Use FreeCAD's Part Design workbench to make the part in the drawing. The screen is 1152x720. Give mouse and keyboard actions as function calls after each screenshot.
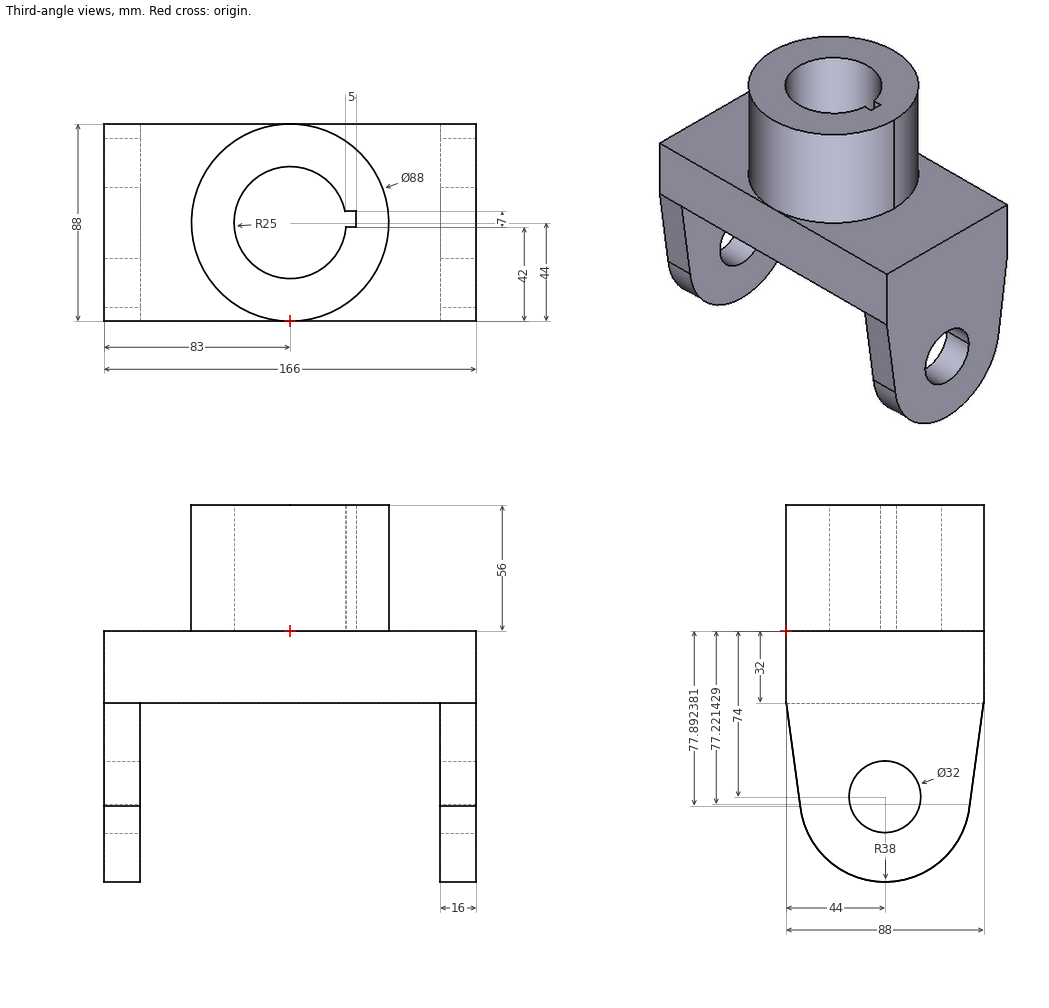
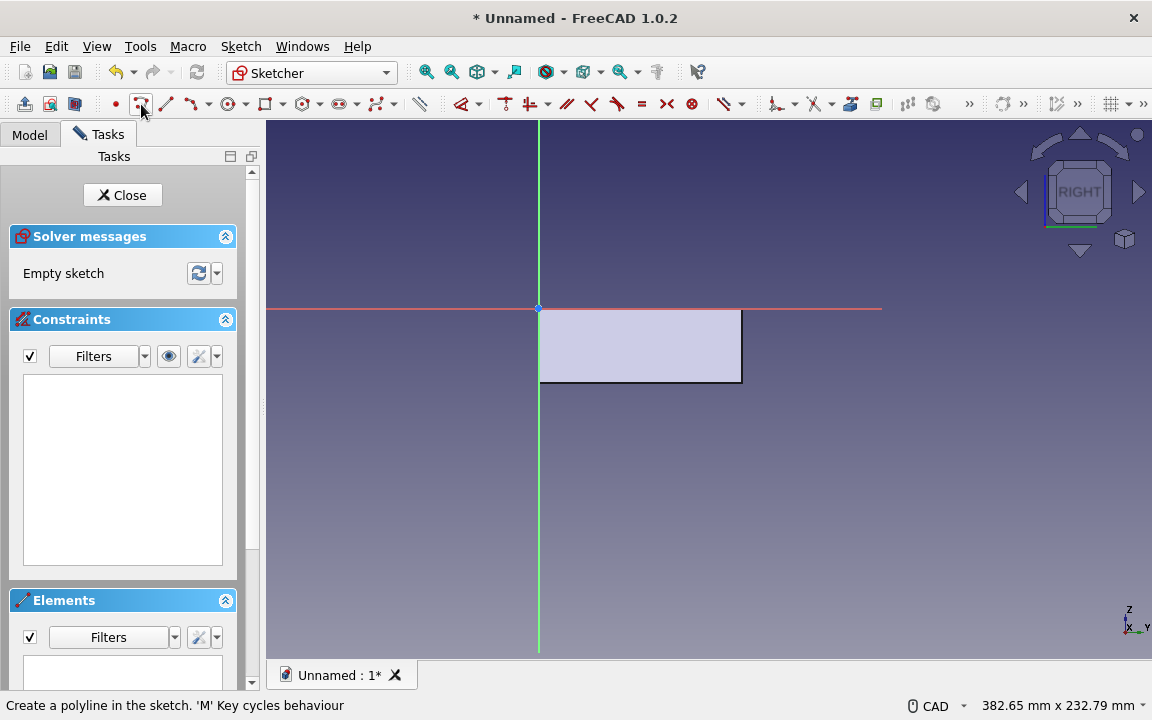
click(728, 487)
click(742, 383)
click(539, 383)
click(553, 489)
right_click(553, 489)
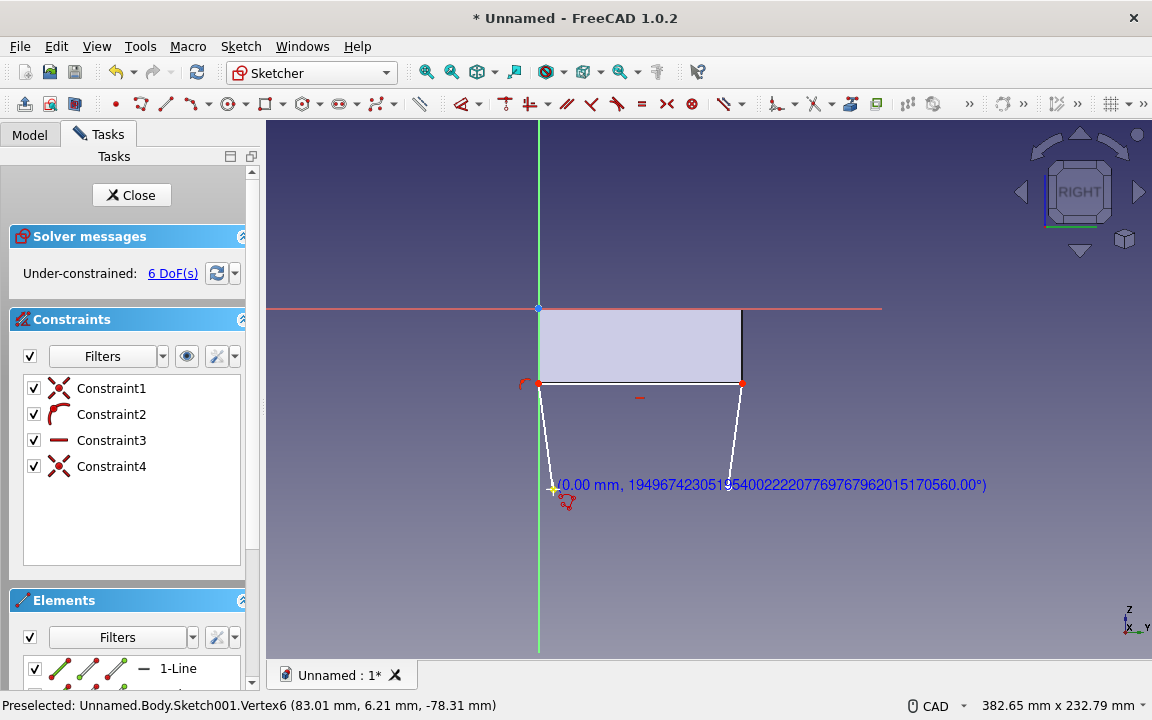
click(190, 104)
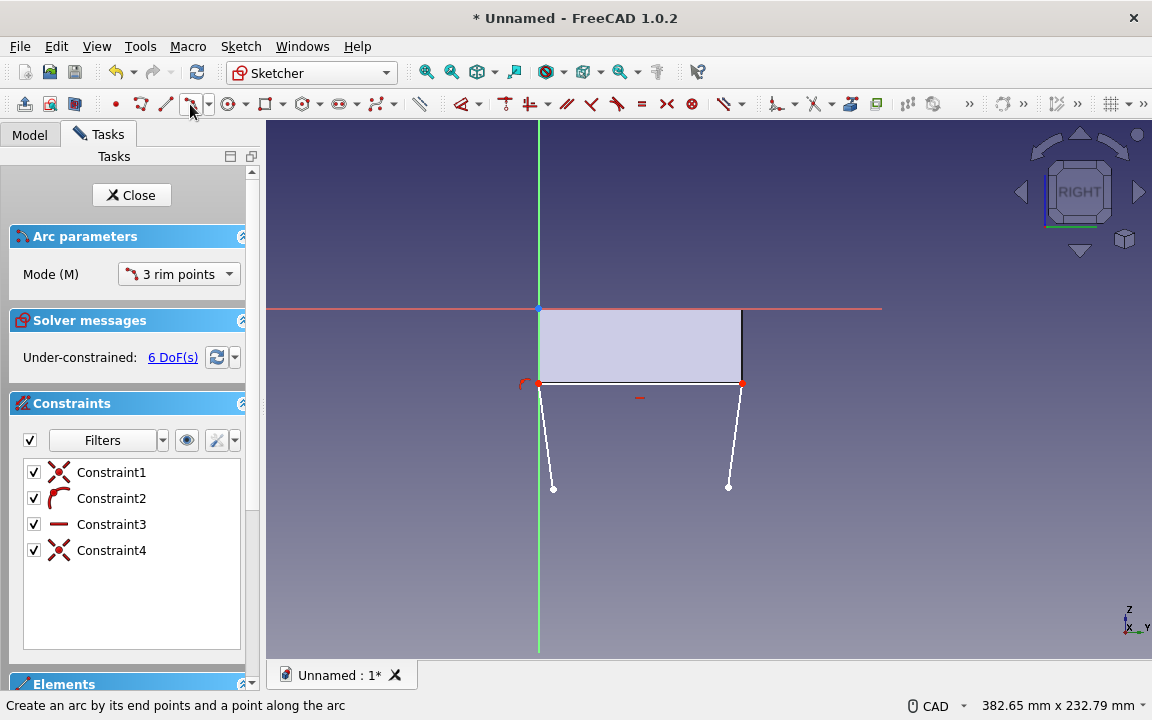
click(553, 490)
click(728, 488)
click(641, 568)
key(Escape)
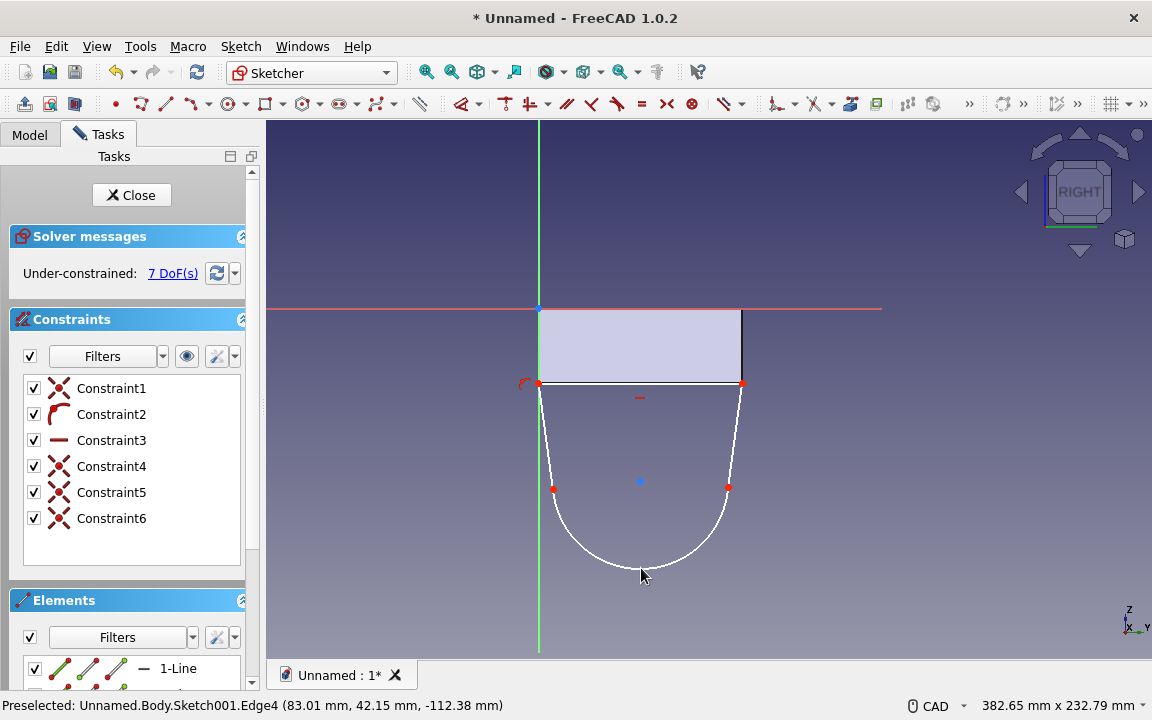
click(460, 104)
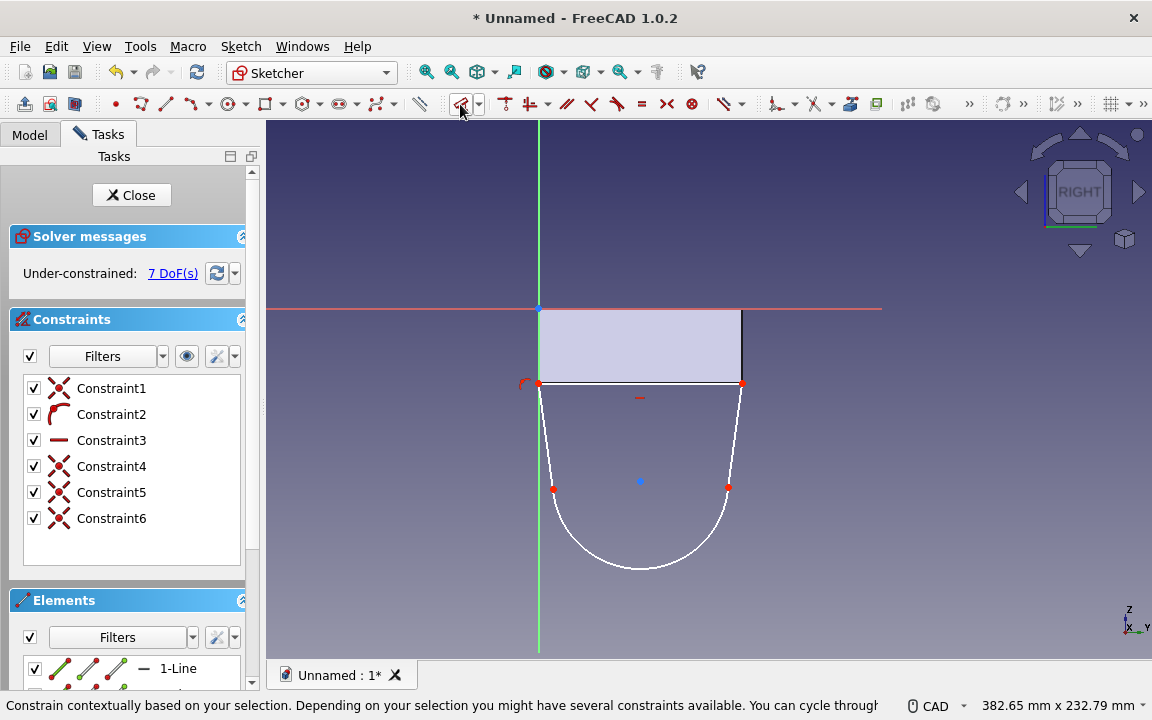
click(592, 555)
click(574, 582)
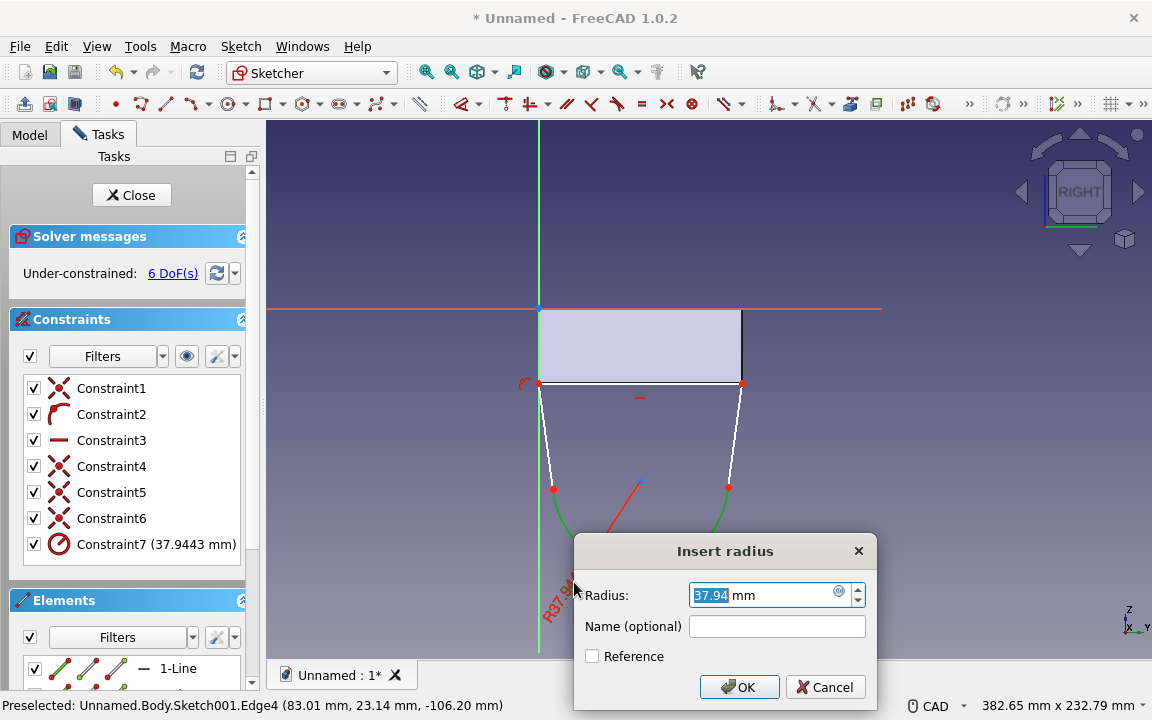
text(38)
key(Return)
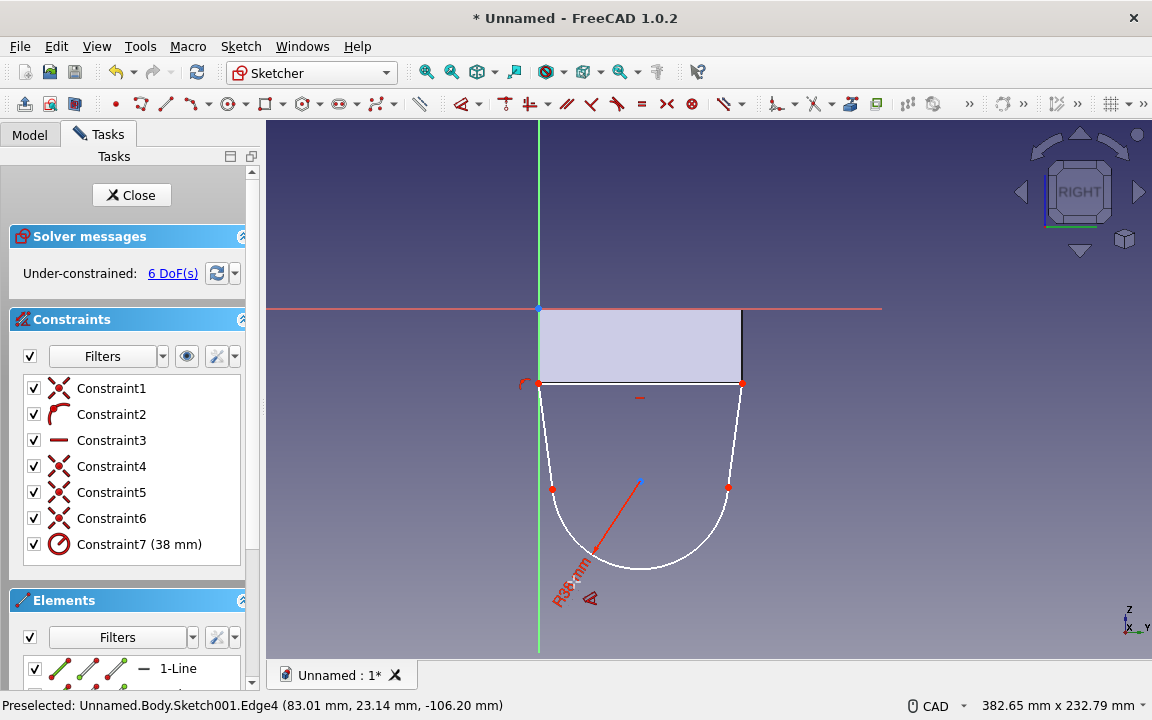
click(681, 384)
click(640, 350)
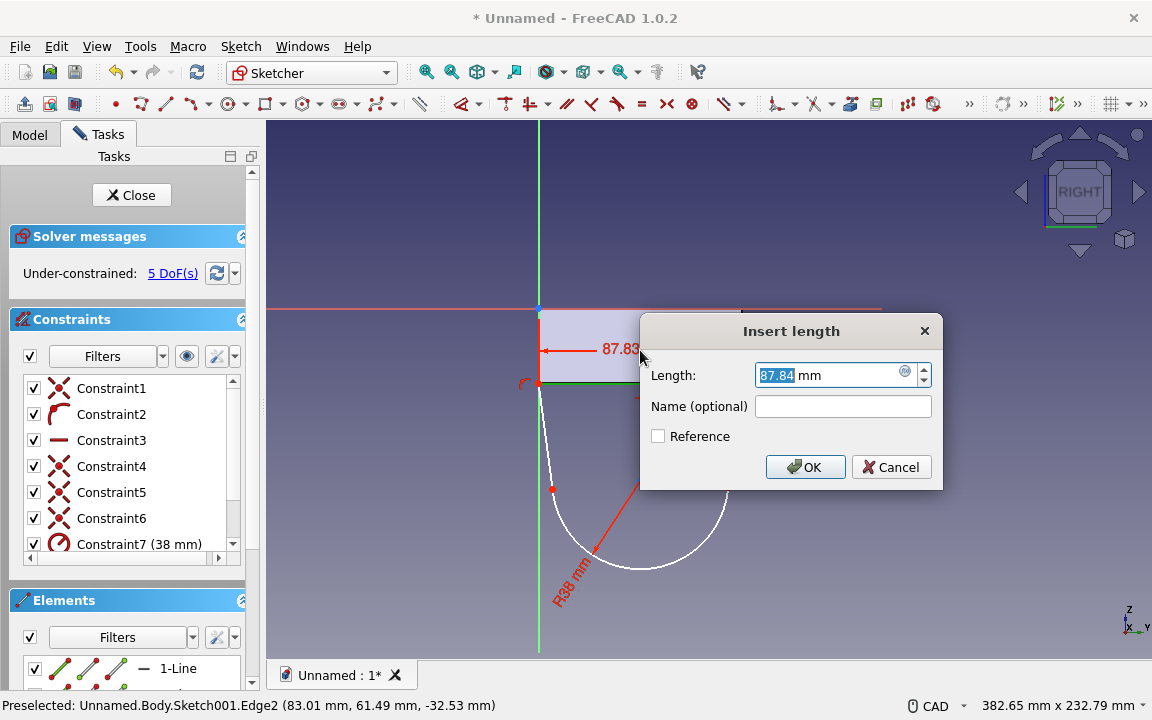
text(88)
key(Return)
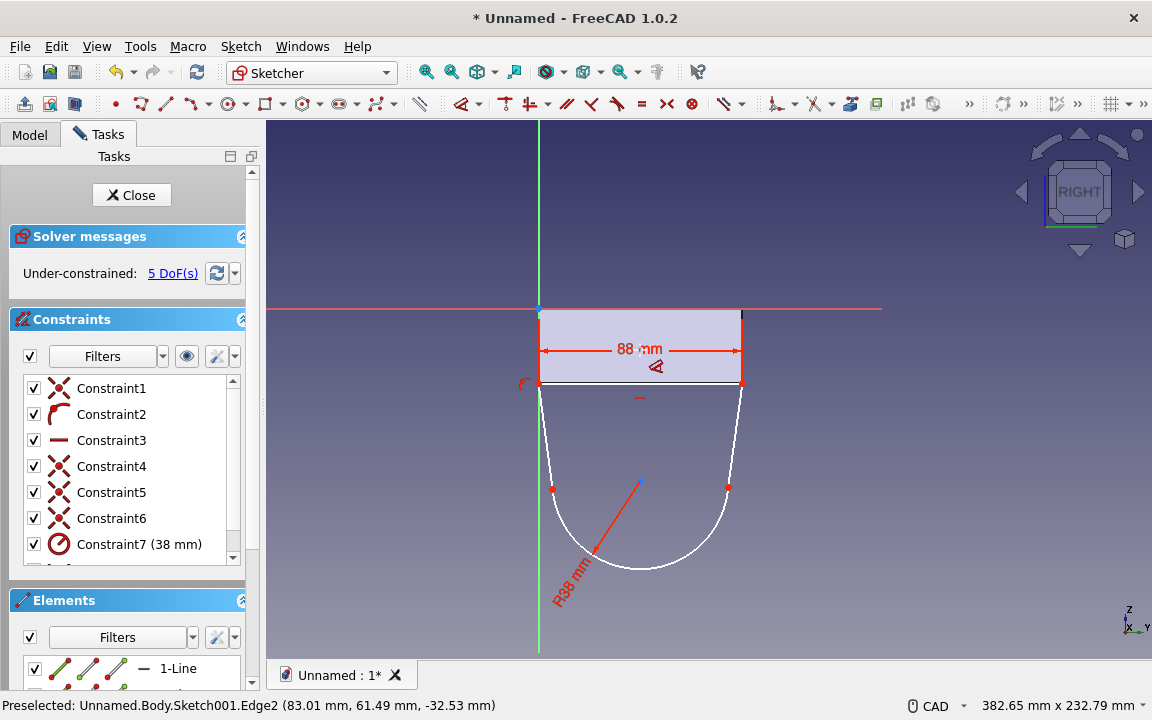
click(742, 384)
click(776, 346)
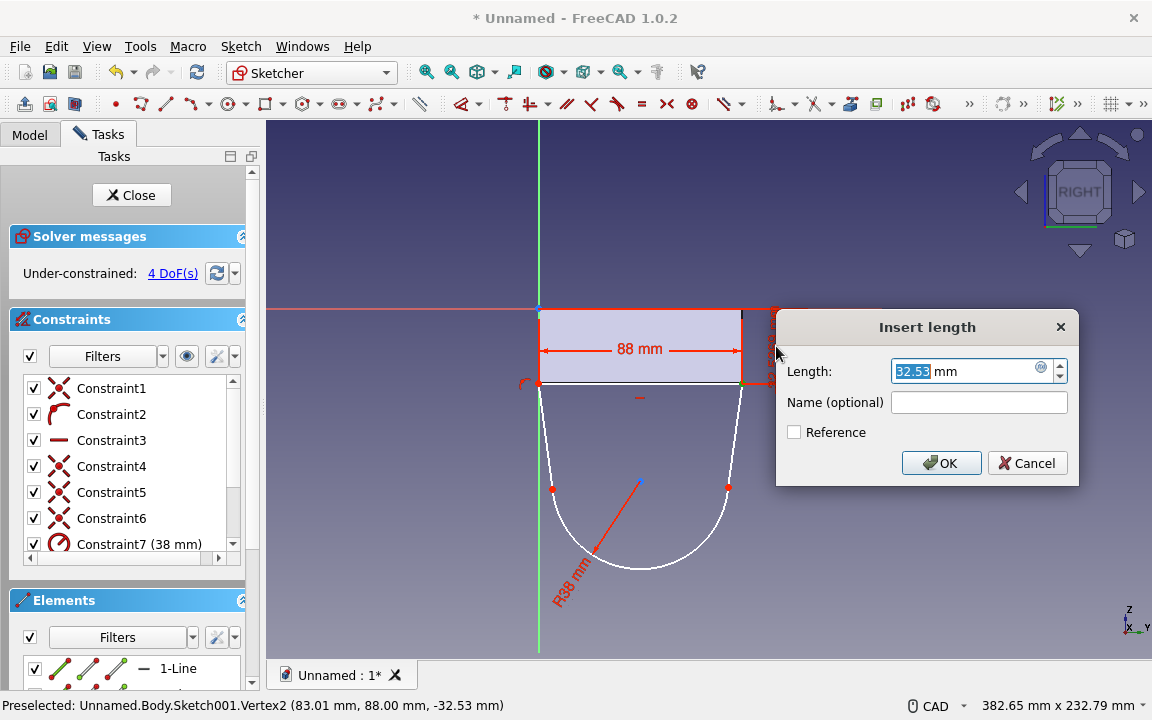
text(32)
key(Return)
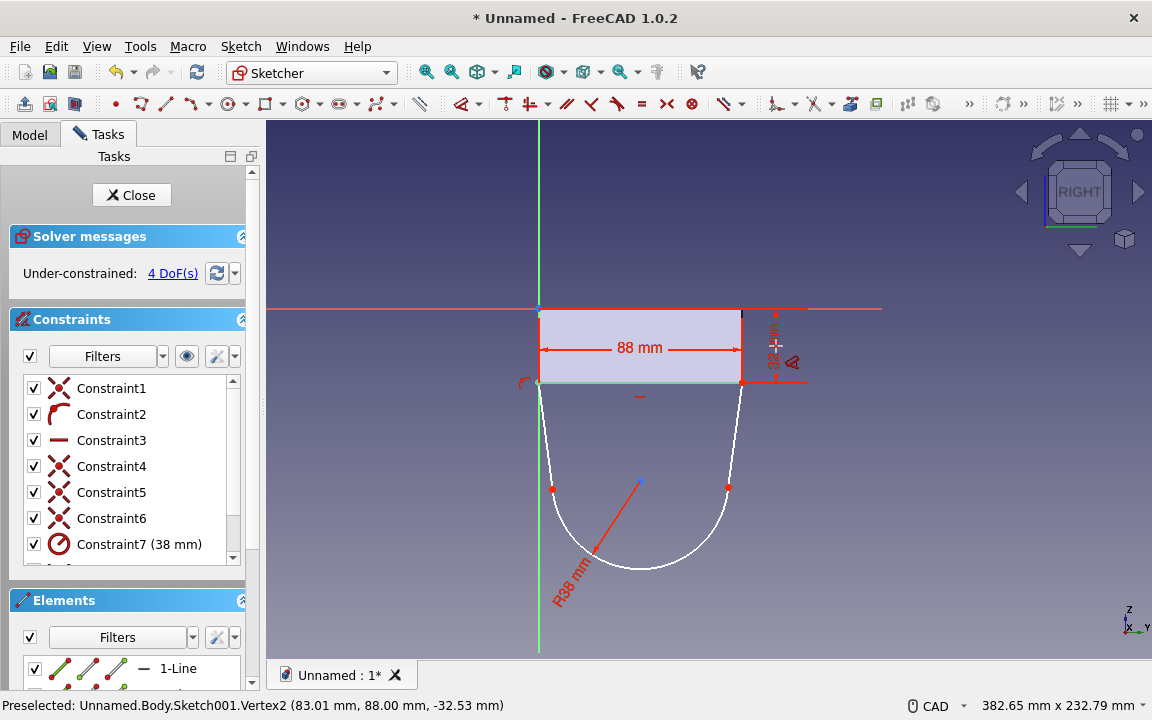
click(640, 481)
click(589, 275)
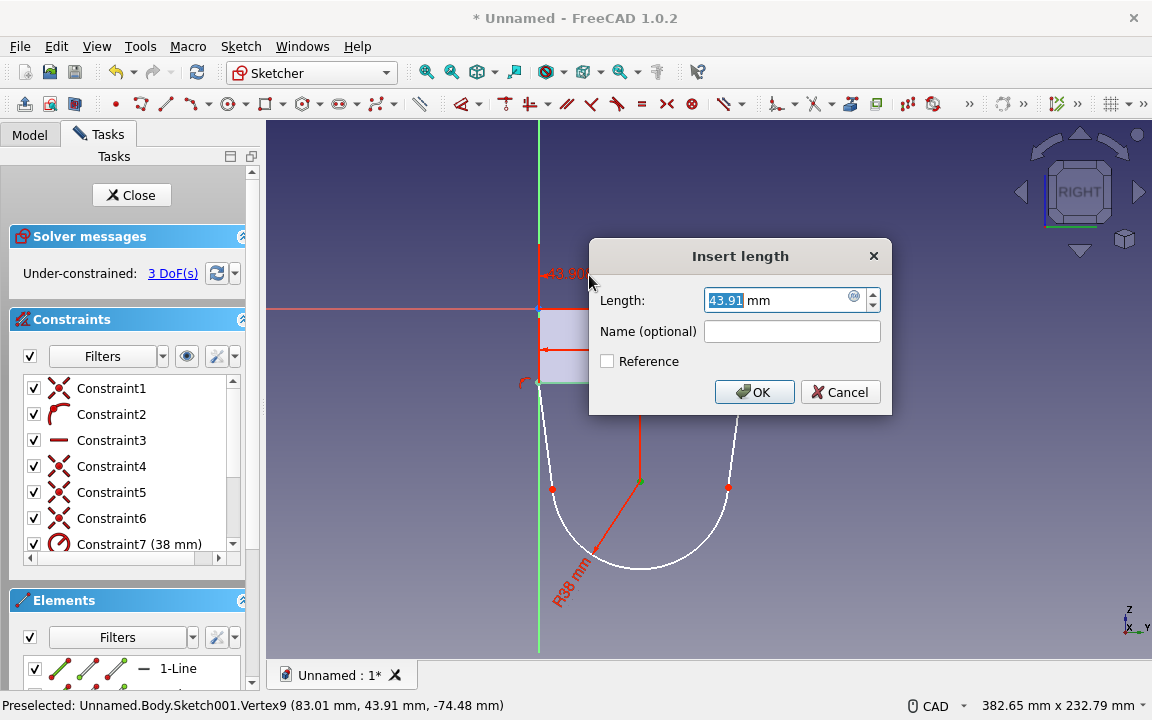
text(44)
key(Return)